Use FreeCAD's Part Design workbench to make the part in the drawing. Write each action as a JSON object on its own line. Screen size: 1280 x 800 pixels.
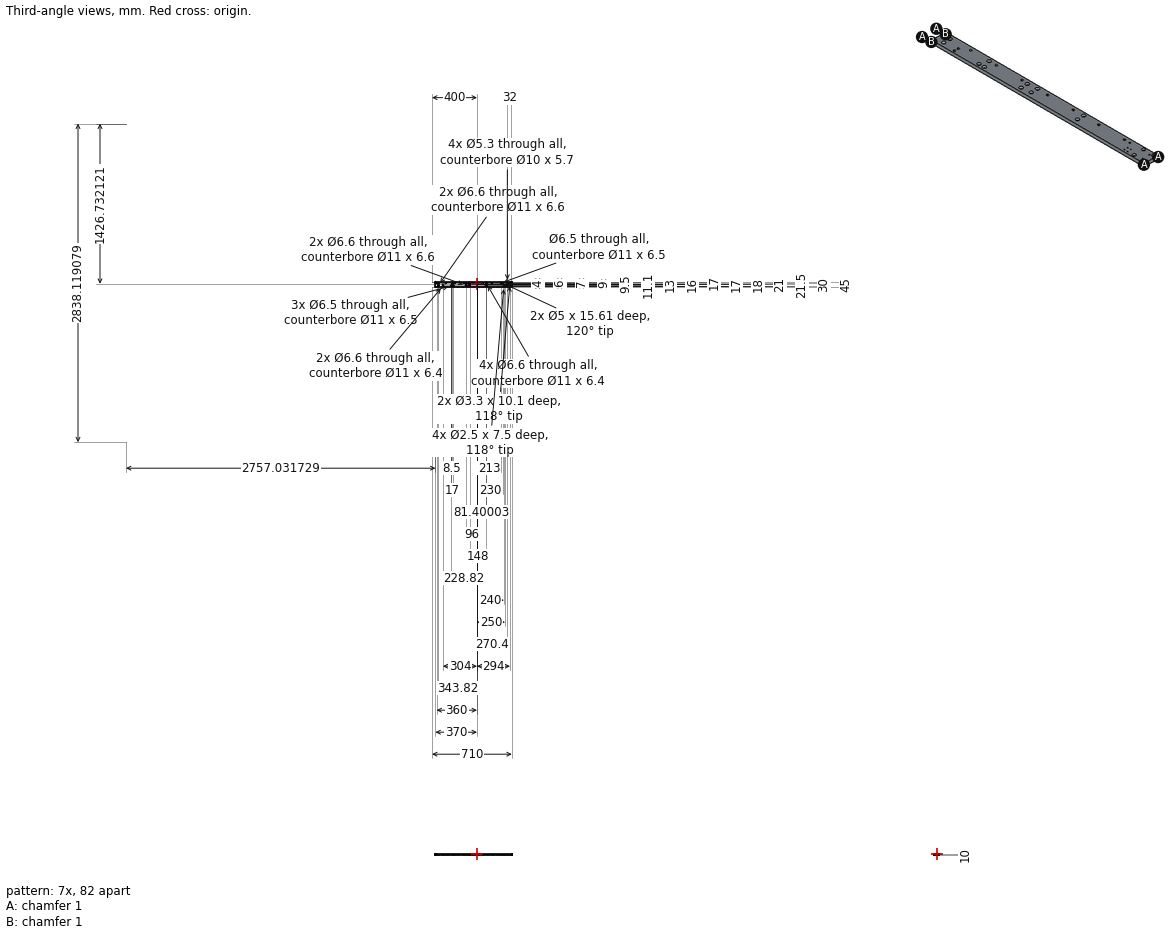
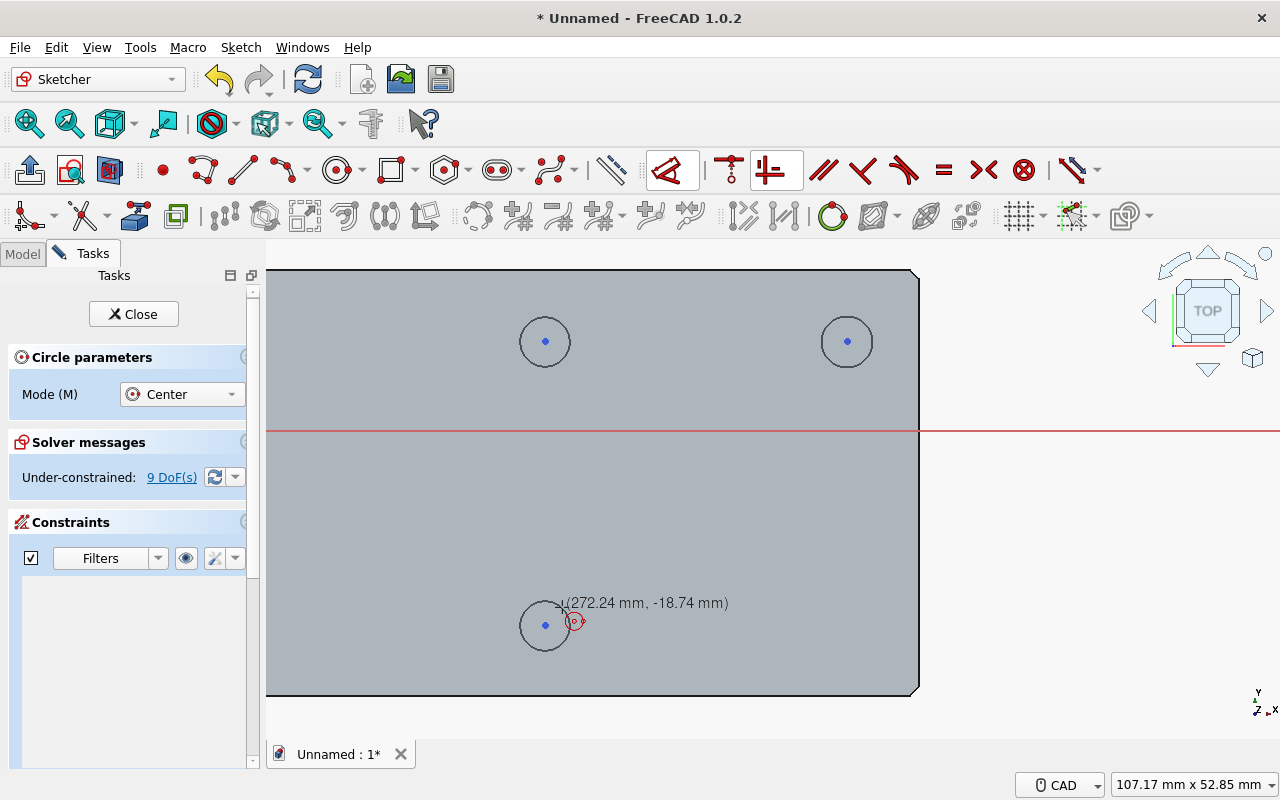
{"action": "left_click", "coordinate": [847, 625]}
{"action": "left_click", "coordinate": [865, 607]}
{"action": "key", "text": "Escape"}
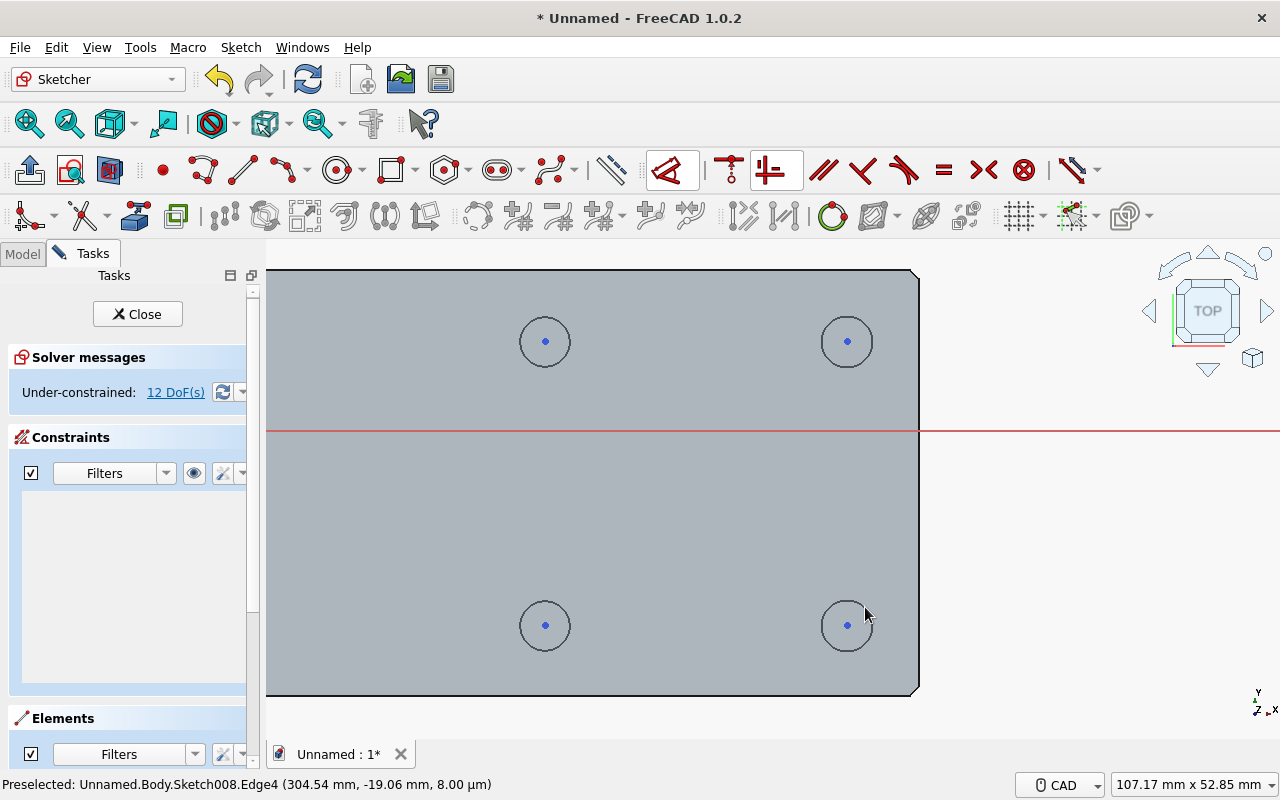
{"action": "left_click", "coordinate": [562, 324]}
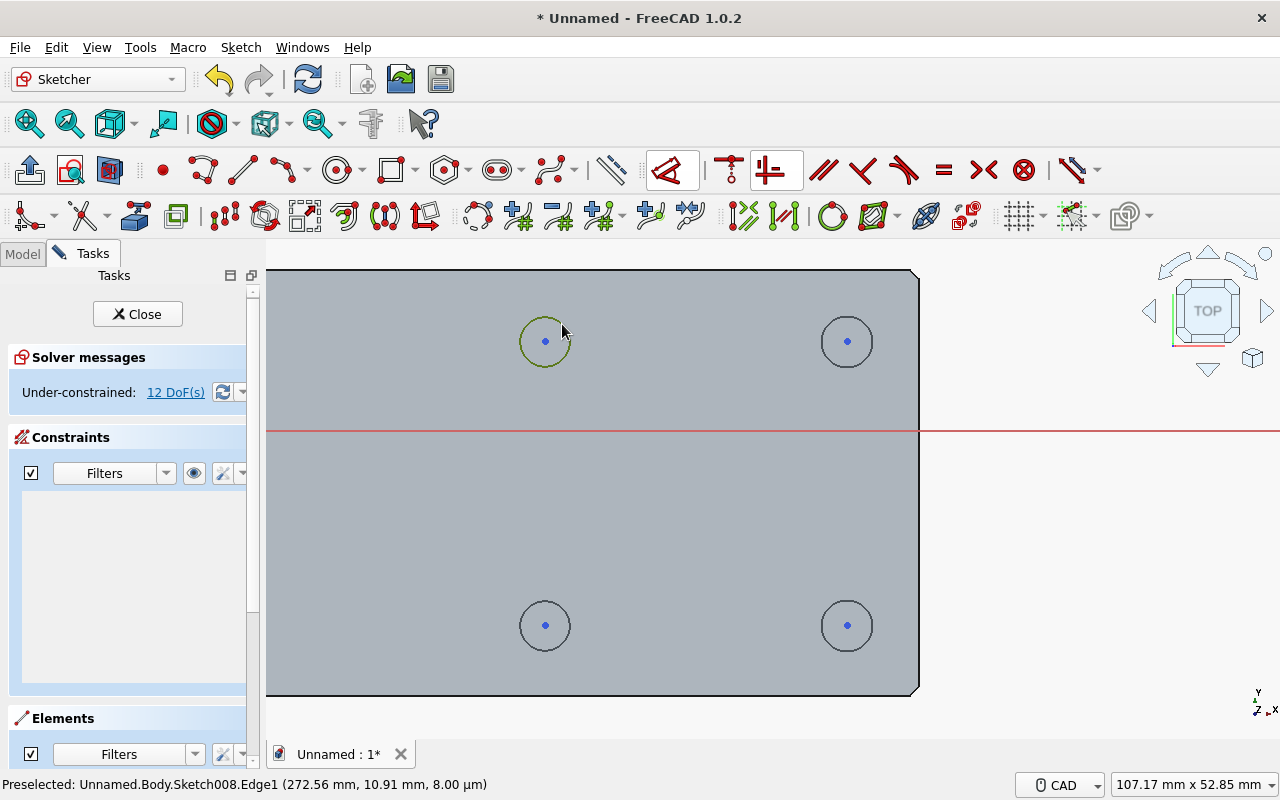
{"action": "left_click", "coordinate": [865, 324]}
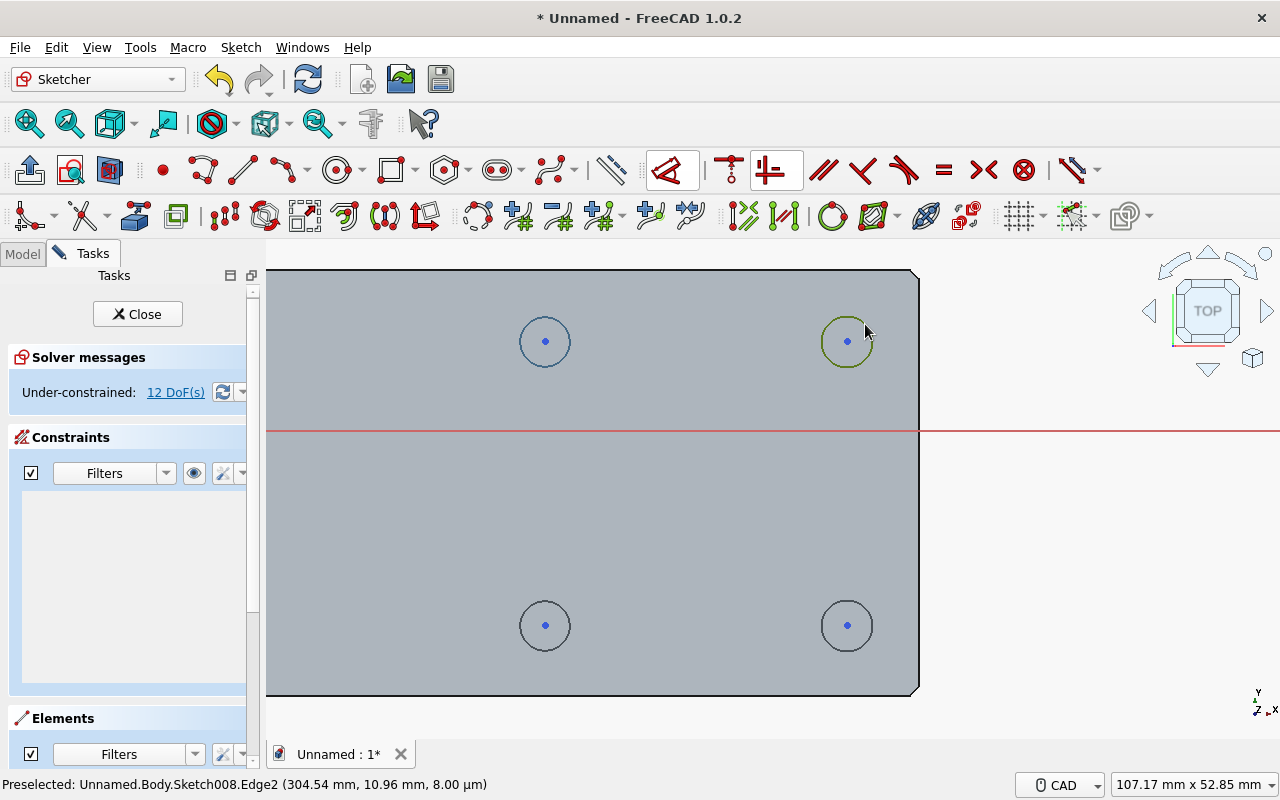
{"action": "left_click", "coordinate": [562, 608]}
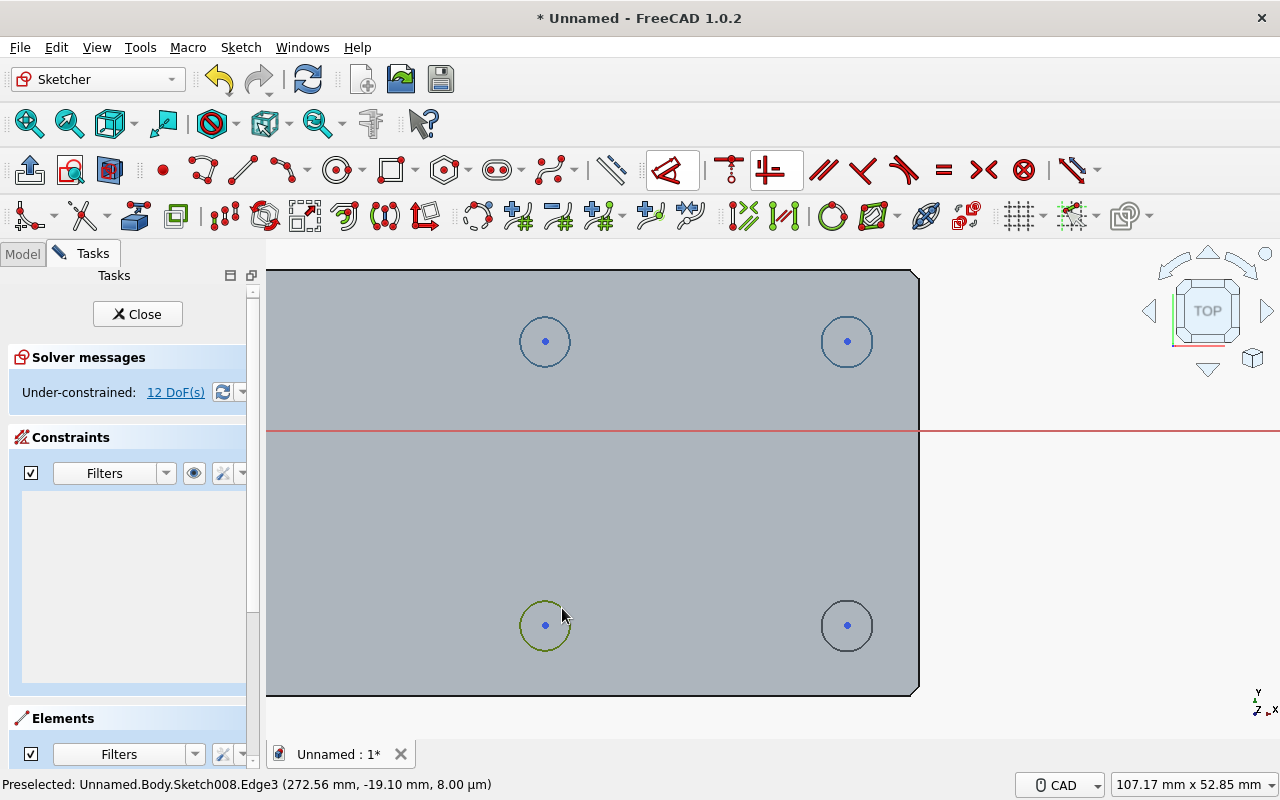
{"action": "left_click", "coordinate": [865, 608]}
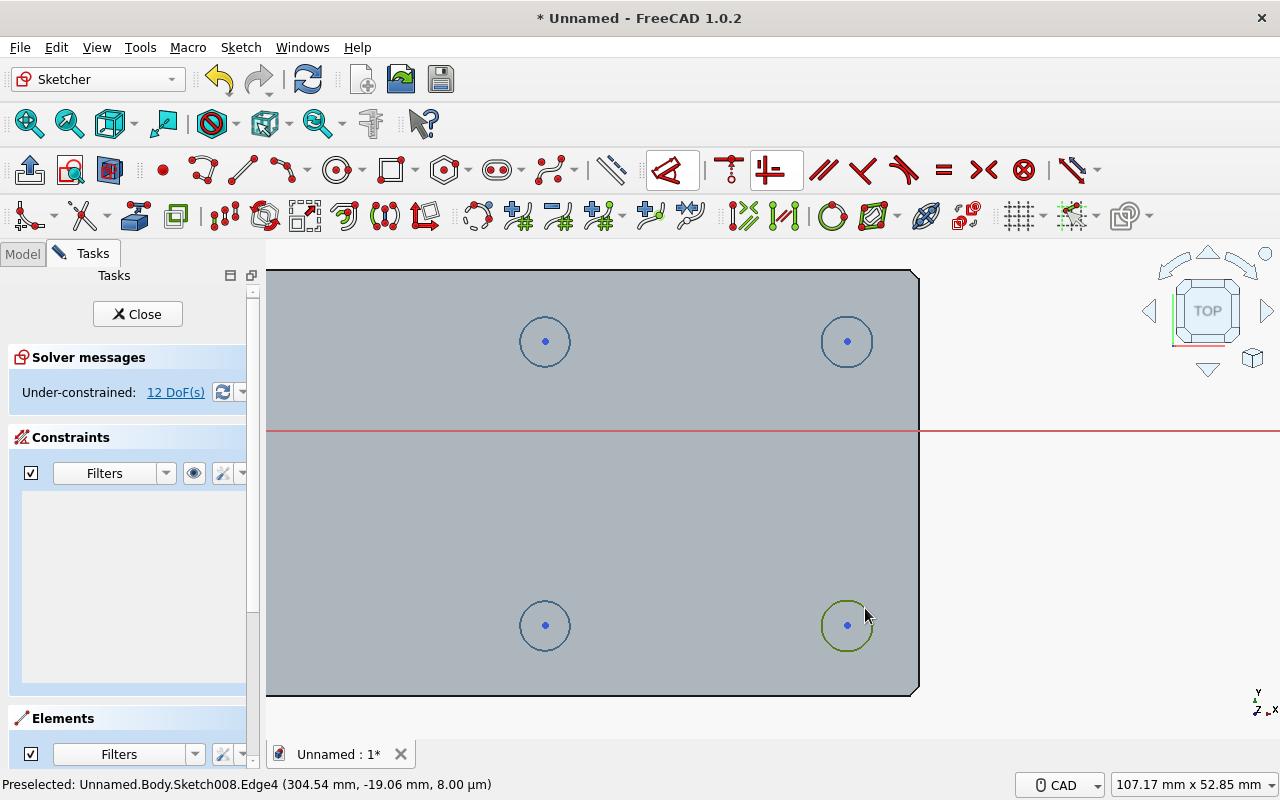
{"action": "left_click", "coordinate": [944, 170]}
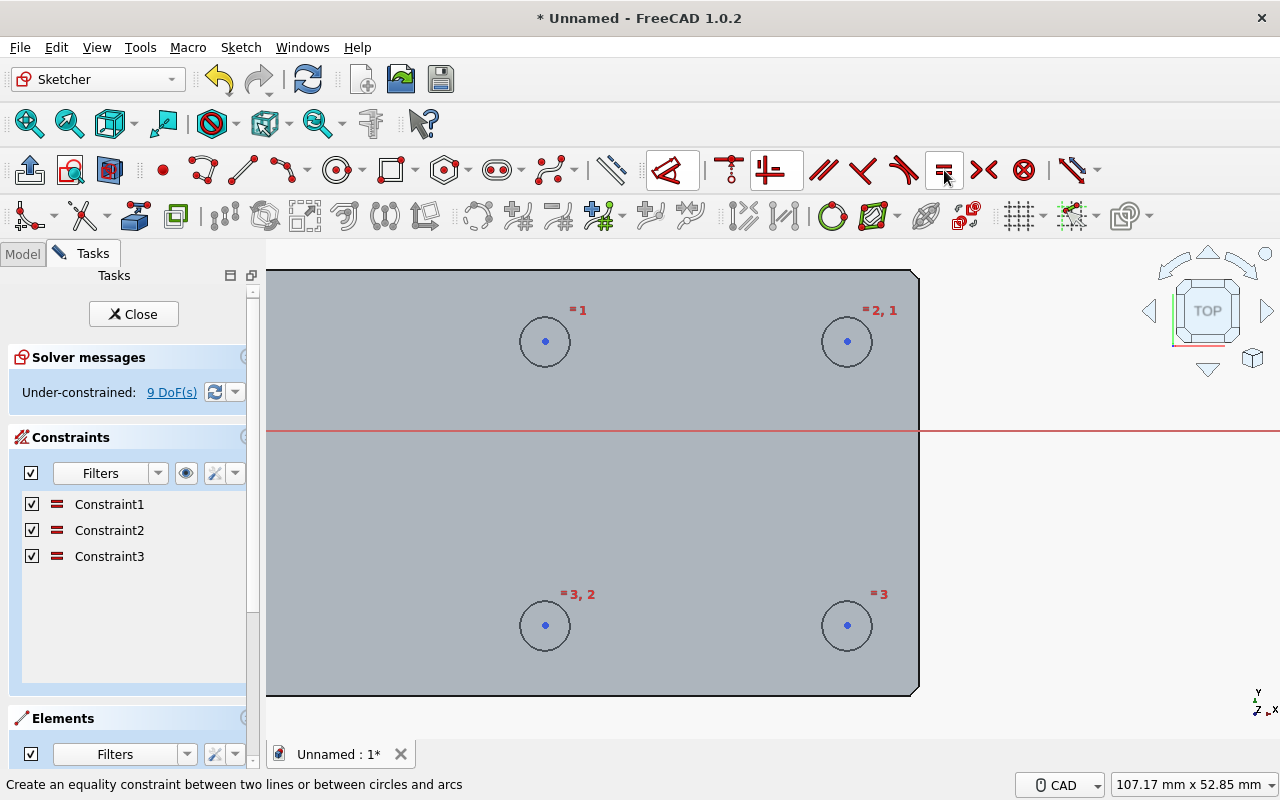
{"action": "left_click", "coordinate": [545, 342]}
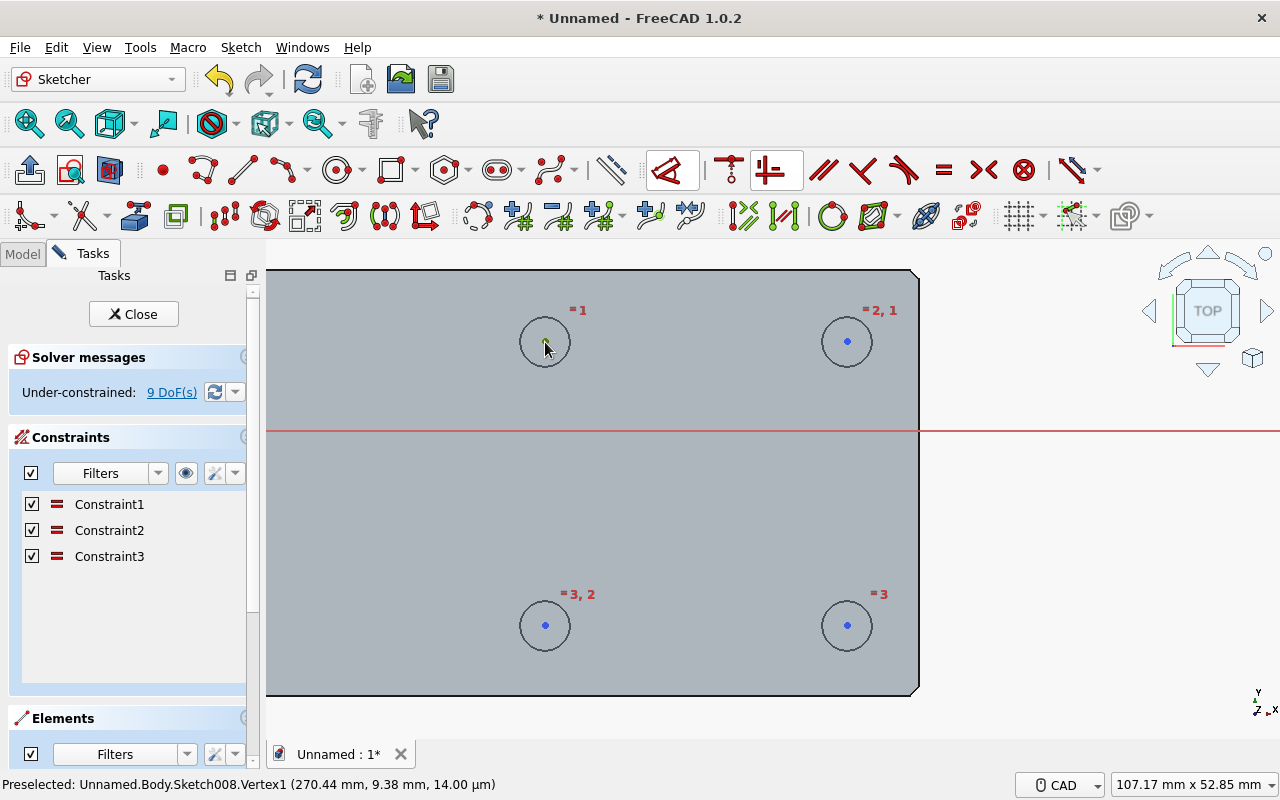
{"action": "left_click", "coordinate": [847, 342]}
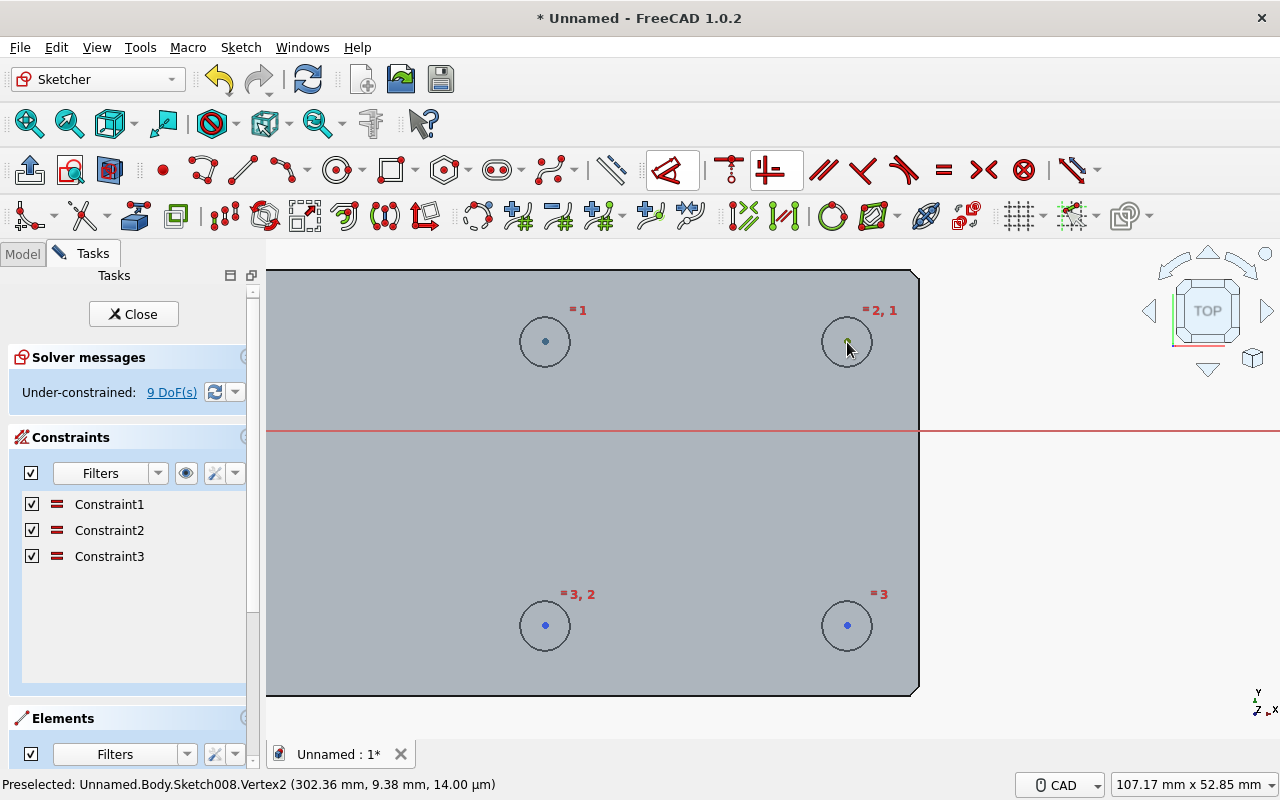
{"action": "key", "text": "h"}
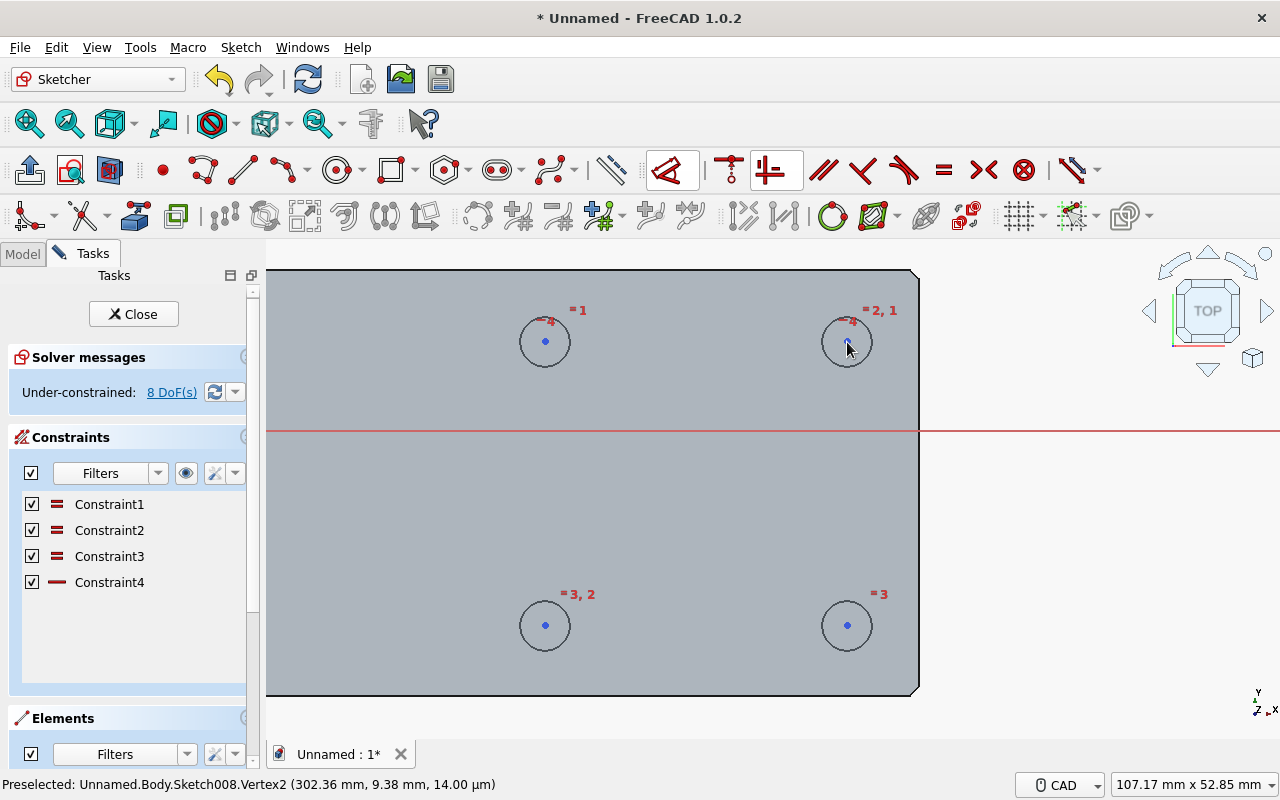
{"action": "left_click", "coordinate": [545, 342]}